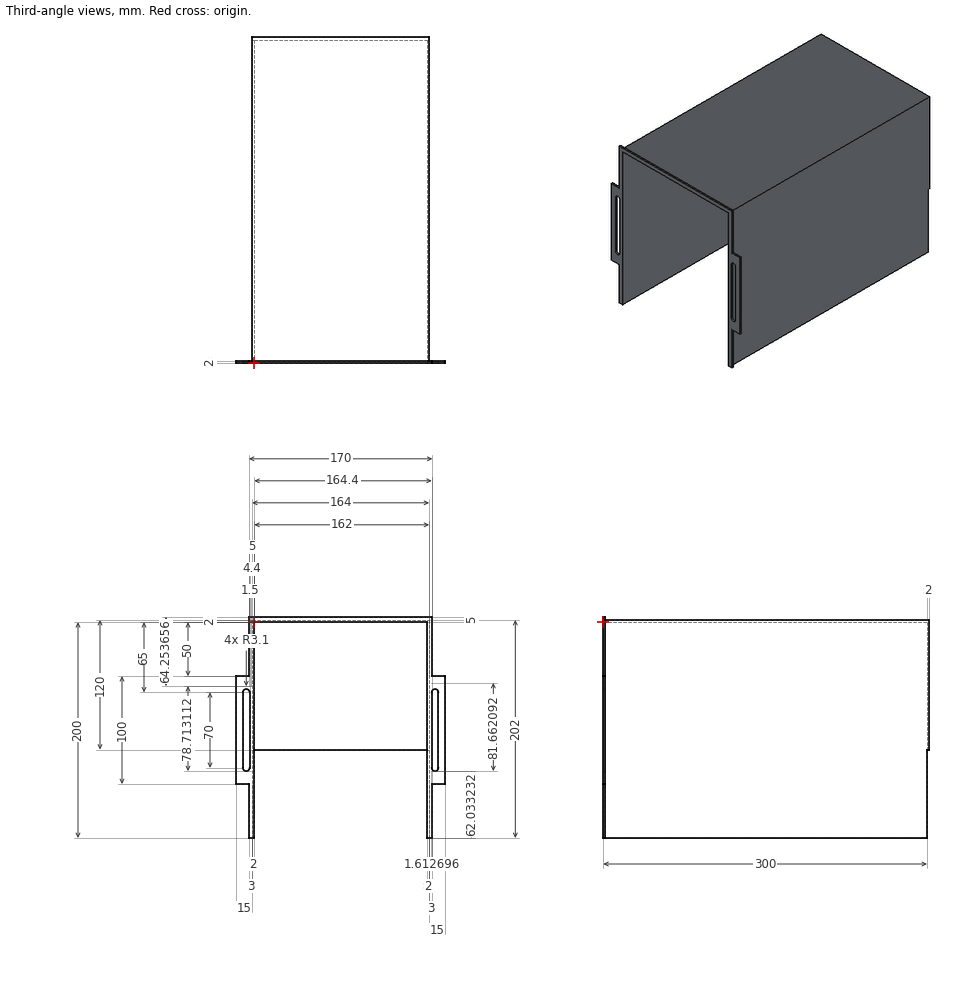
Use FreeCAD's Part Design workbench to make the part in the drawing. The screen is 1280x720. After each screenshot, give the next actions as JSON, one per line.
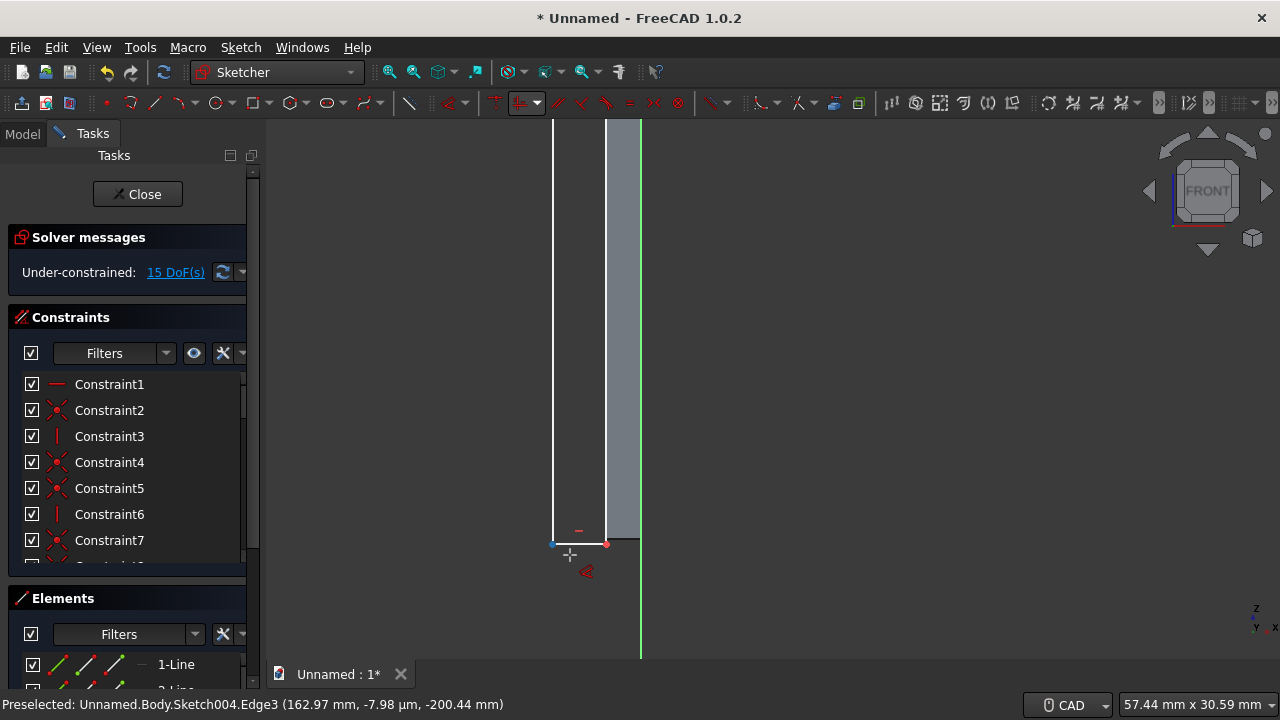
{"action": "left_click", "coordinate": [569, 544]}
{"action": "left_click", "coordinate": [580, 578]}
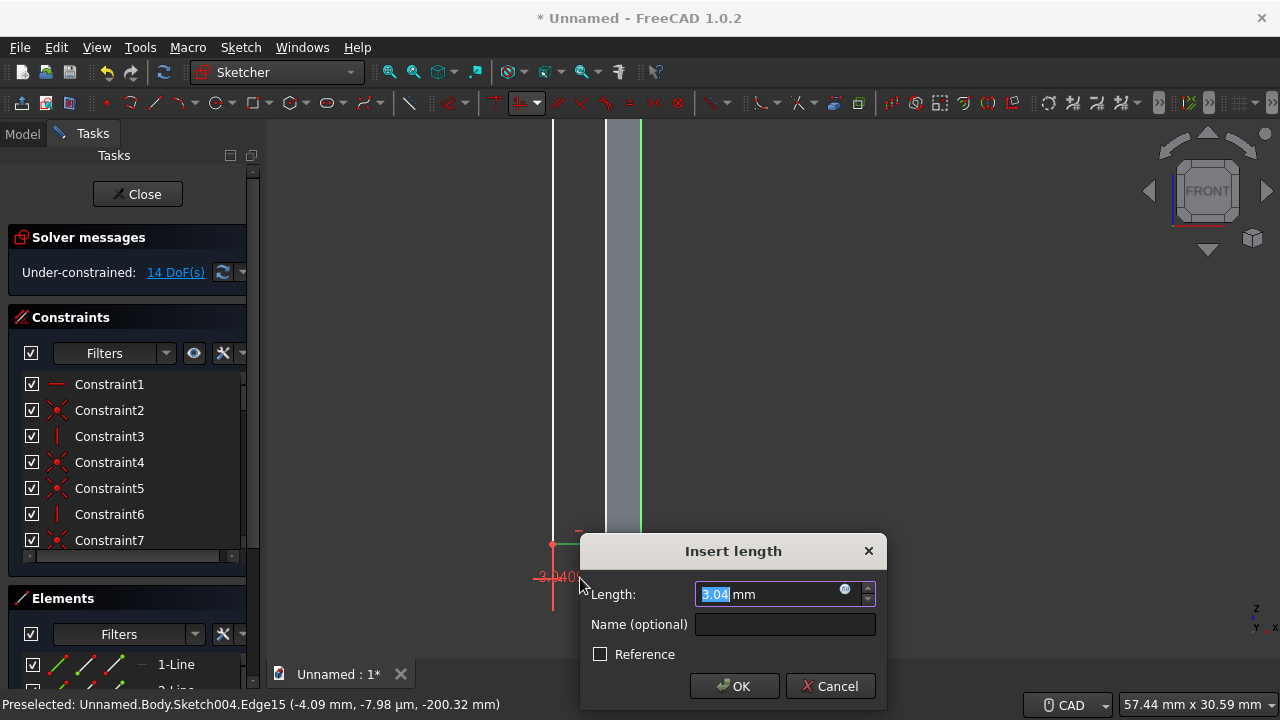
{"action": "type", "text": "3"}
{"action": "key", "text": "Return"}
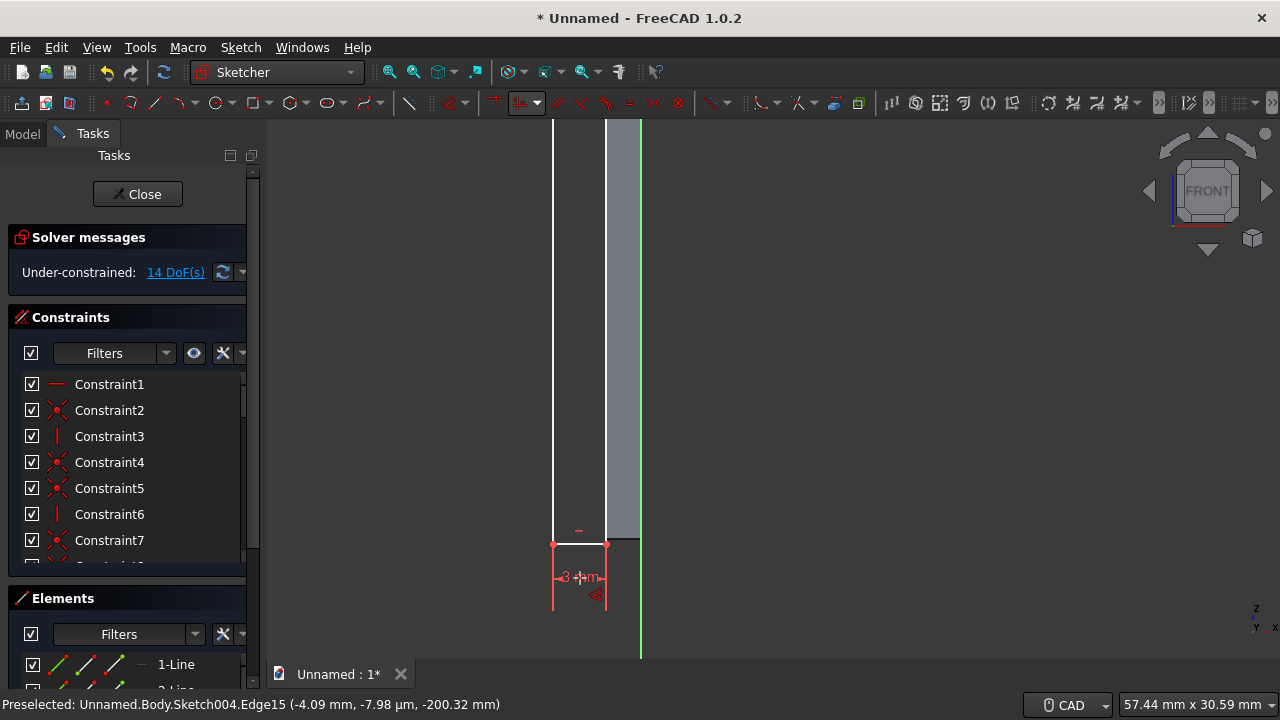
{"action": "scroll", "coordinate": [570, 555], "scroll_direction": "down", "scroll_amount": 12}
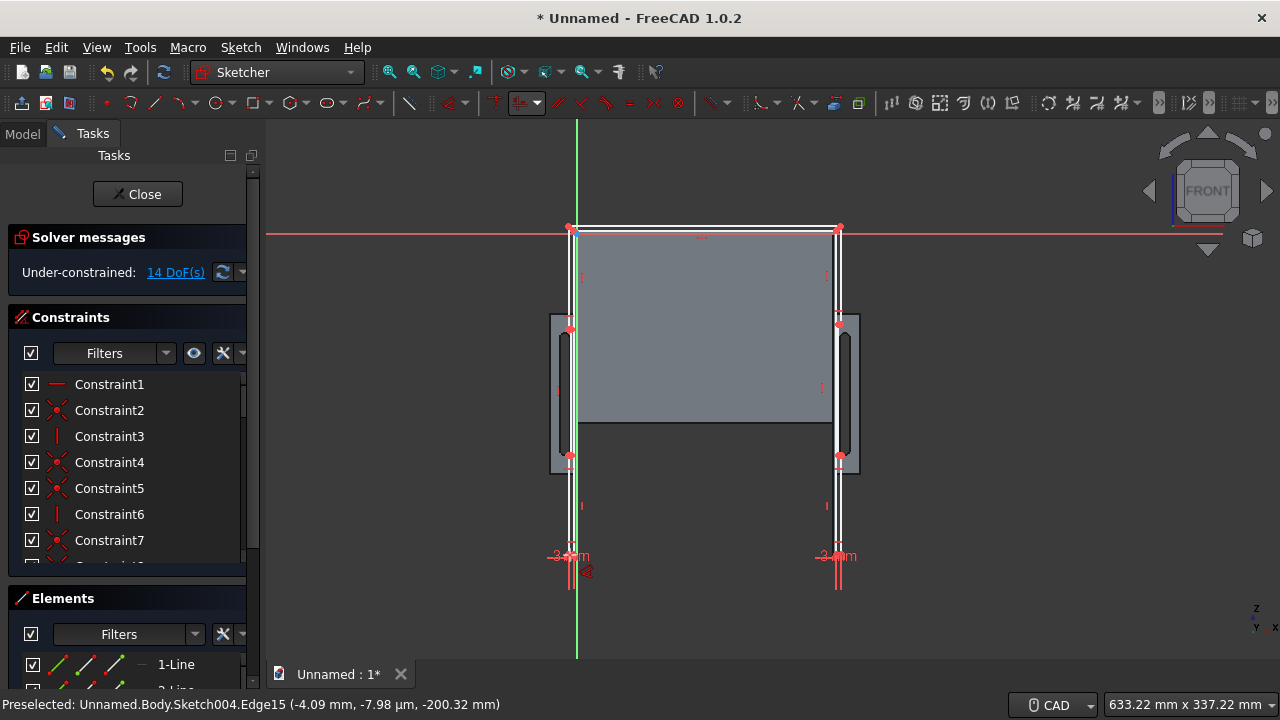
{"action": "scroll", "coordinate": [574, 231], "scroll_direction": "up", "scroll_amount": 13}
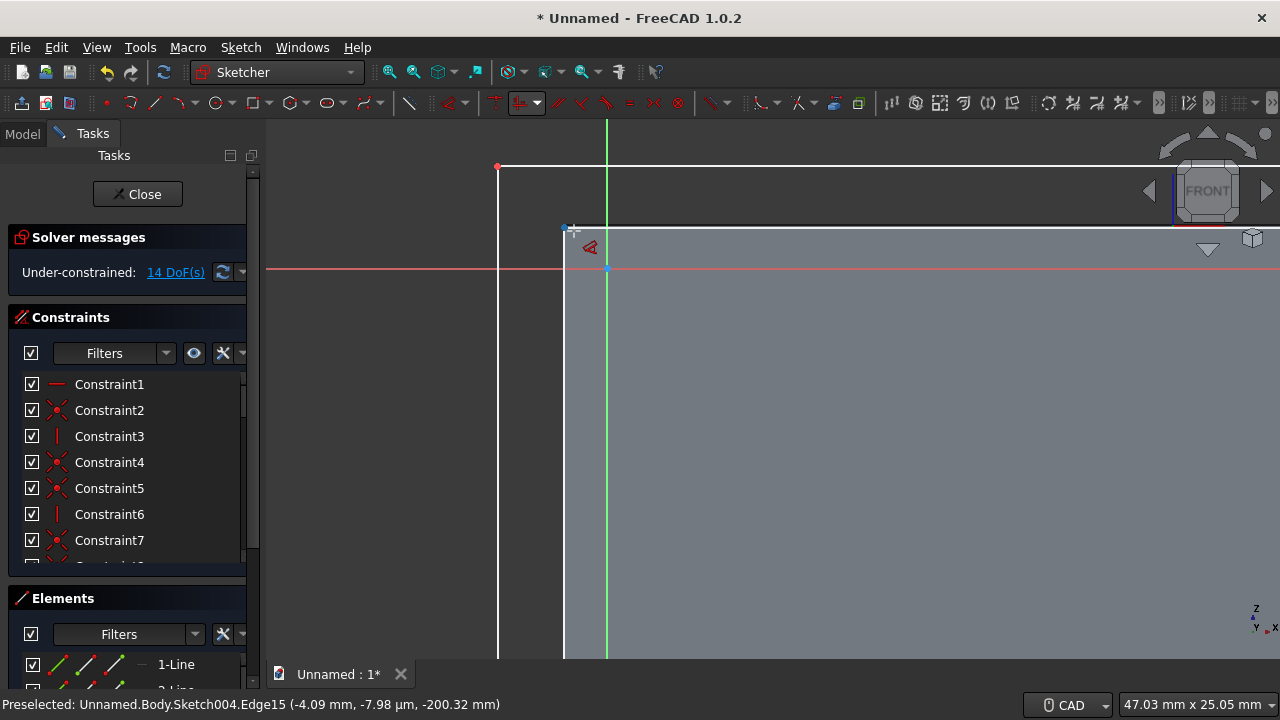
{"action": "left_click", "coordinate": [564, 228]}
{"action": "left_click", "coordinate": [586, 194]}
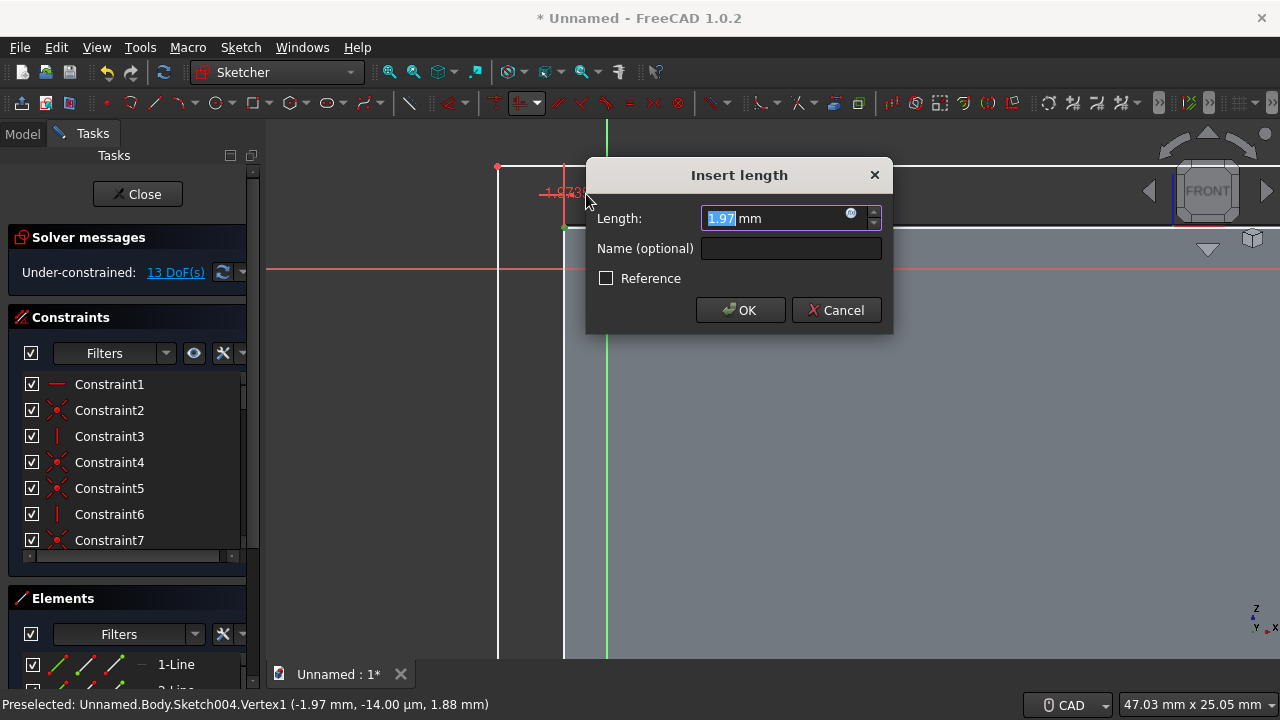
{"action": "type", "text": "2"}
{"action": "key", "text": "Return"}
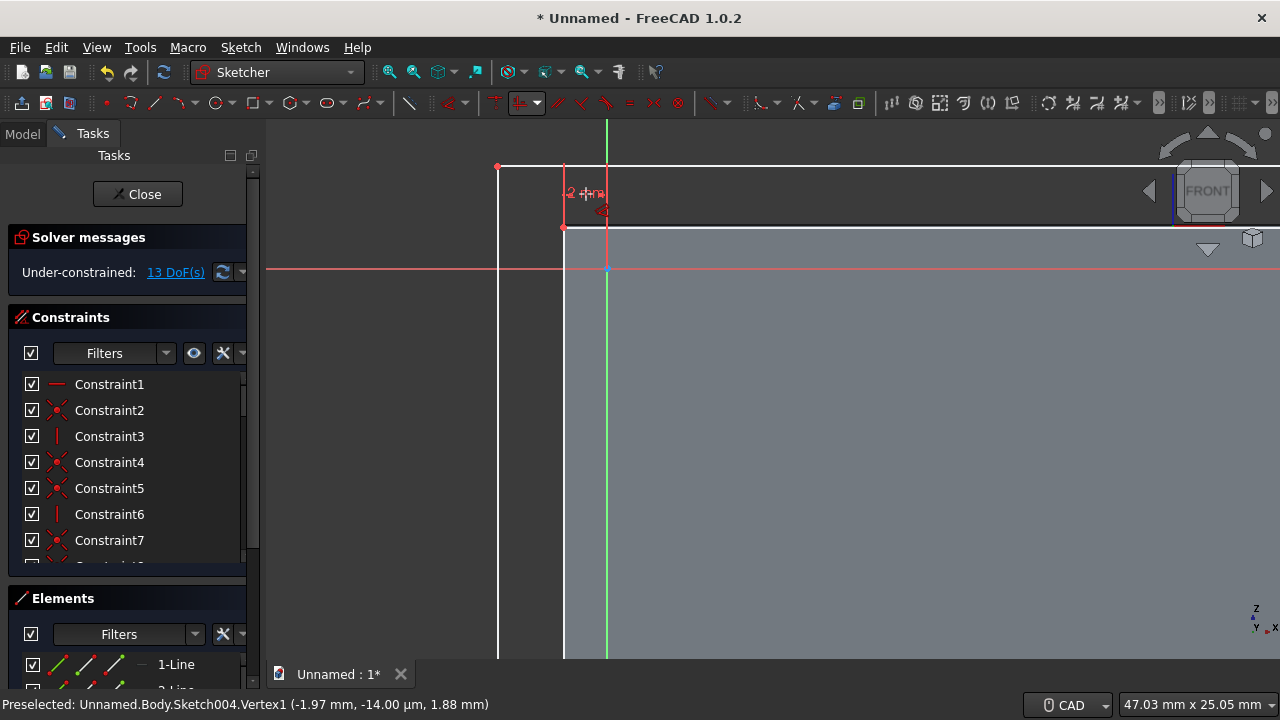
{"action": "left_click", "coordinate": [564, 228]}
{"action": "left_click", "coordinate": [530, 248]}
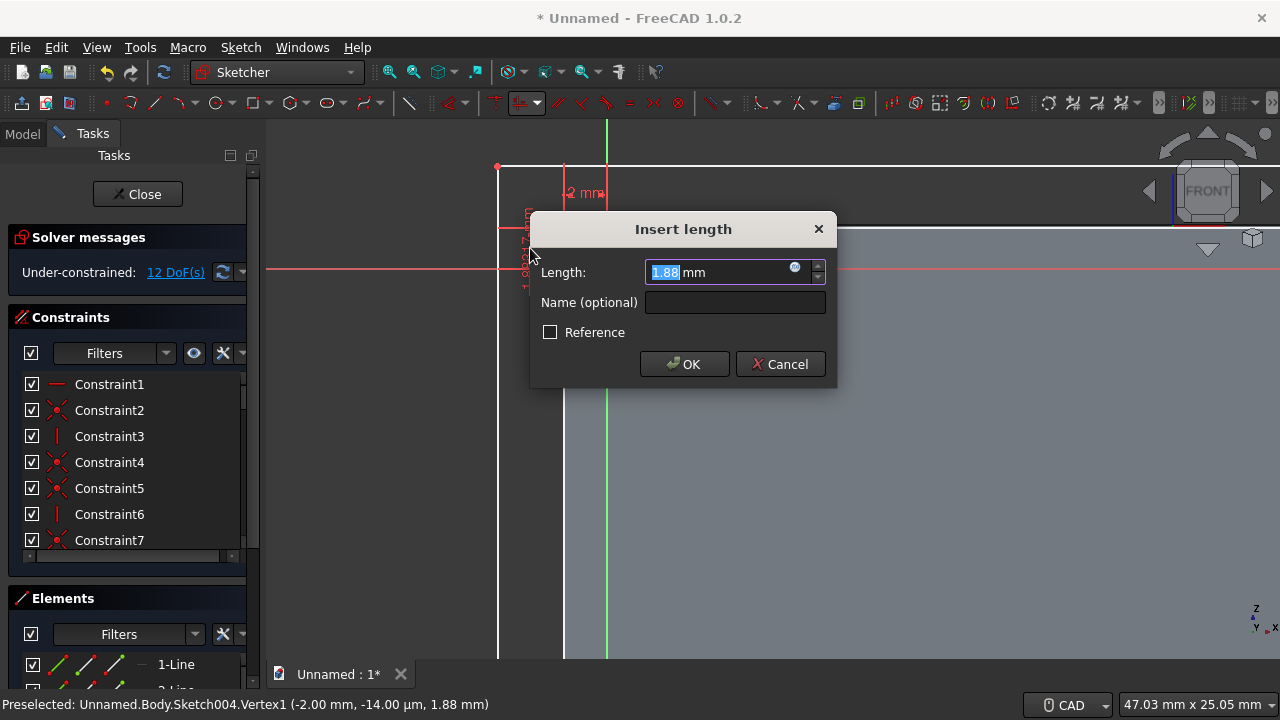
{"action": "type", "text": "2"}
{"action": "key", "text": "Return"}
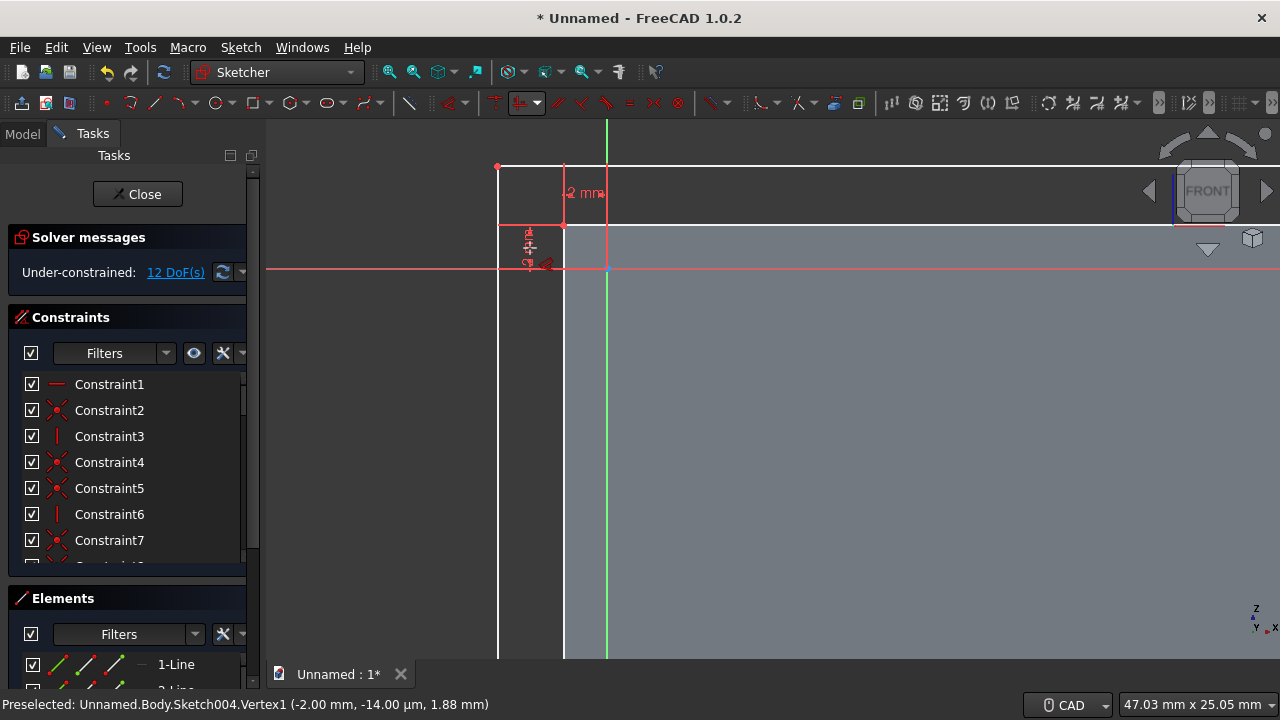
{"action": "scroll", "coordinate": [574, 230], "scroll_direction": "down", "scroll_amount": 13}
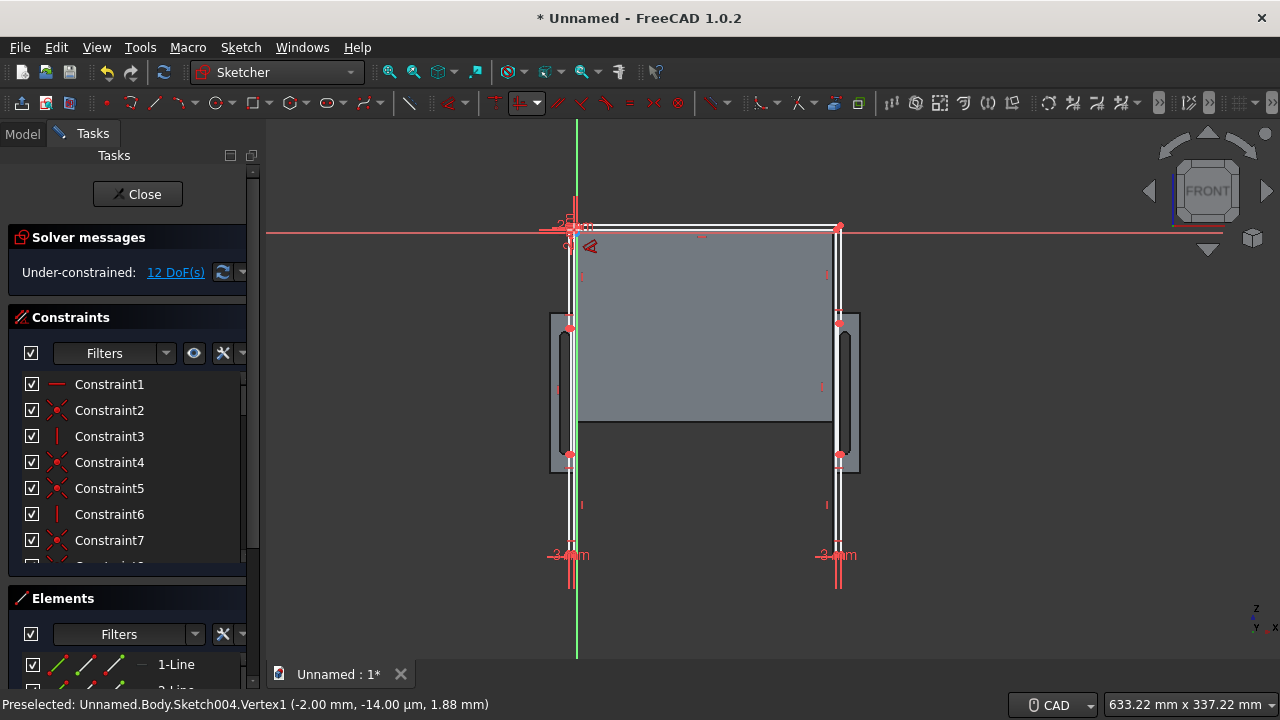
{"action": "scroll", "coordinate": [841, 225], "scroll_direction": "up", "scroll_amount": 9}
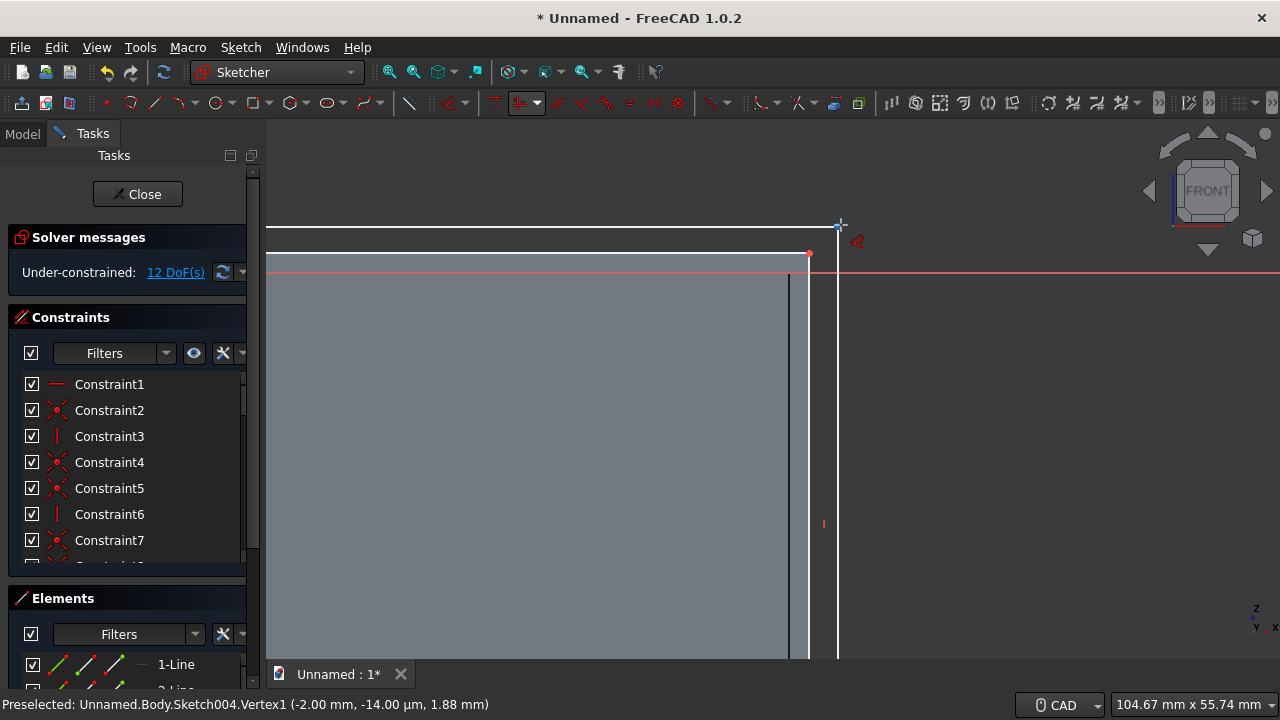
{"action": "left_click", "coordinate": [838, 227]}
{"action": "left_click", "coordinate": [872, 250]}